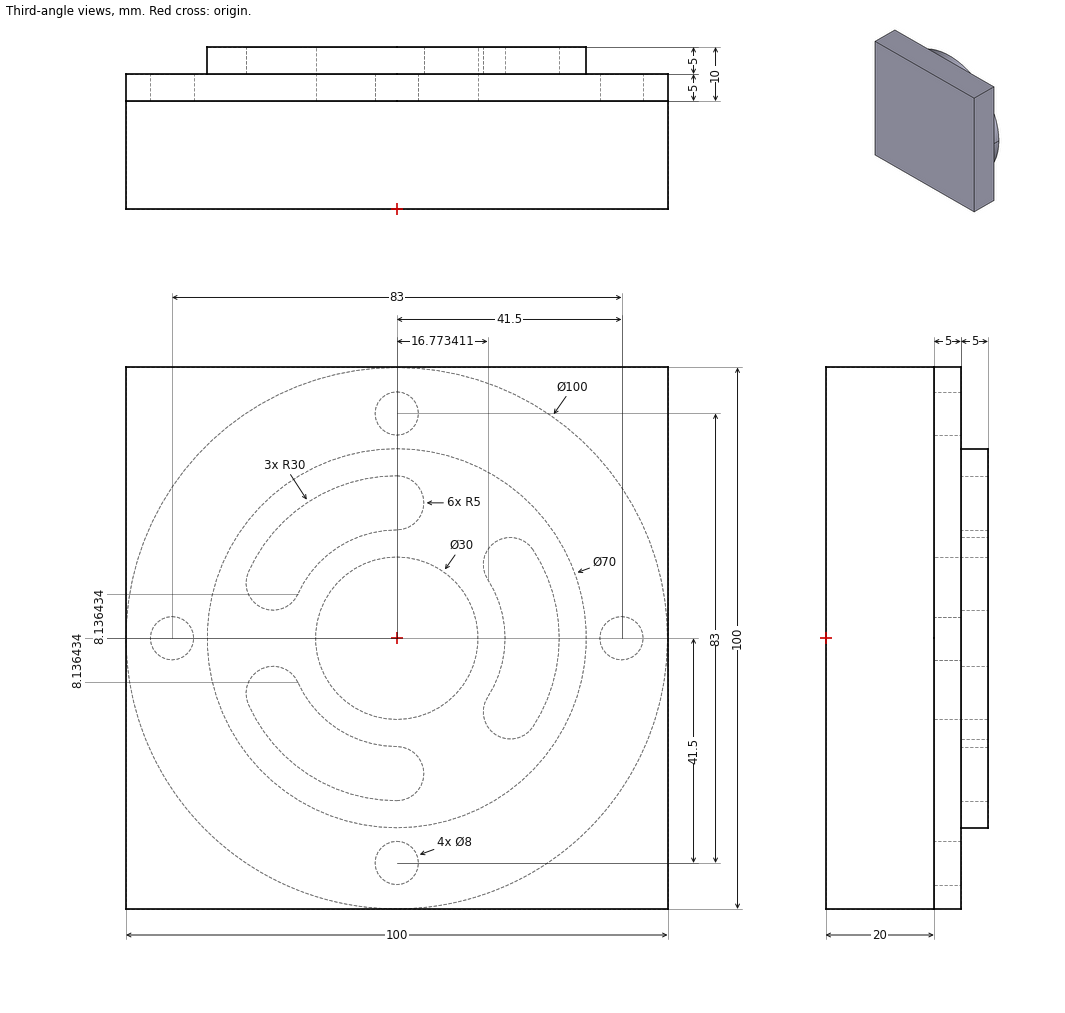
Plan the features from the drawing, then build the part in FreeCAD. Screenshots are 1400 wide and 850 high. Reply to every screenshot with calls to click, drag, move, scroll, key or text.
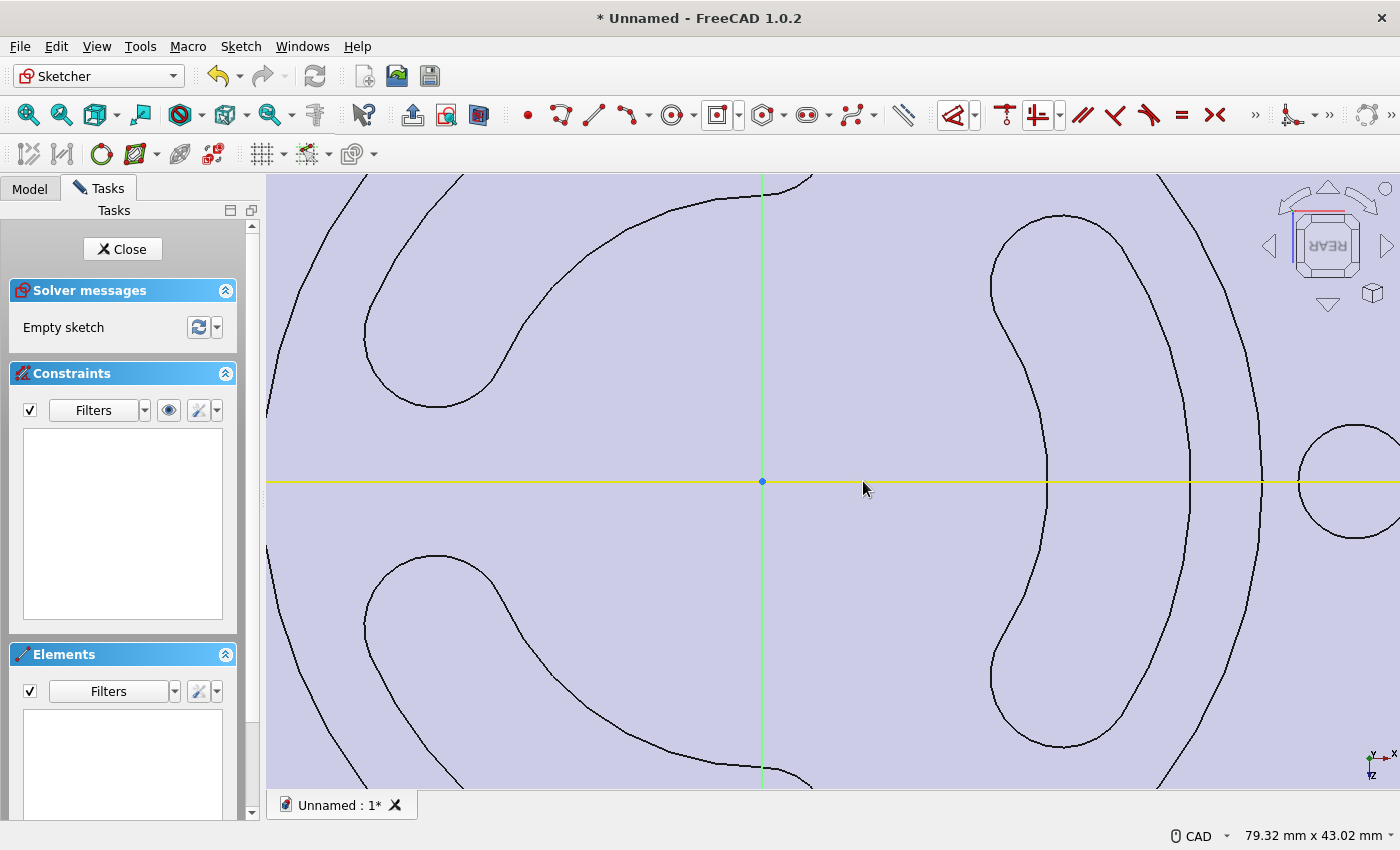
click(672, 116)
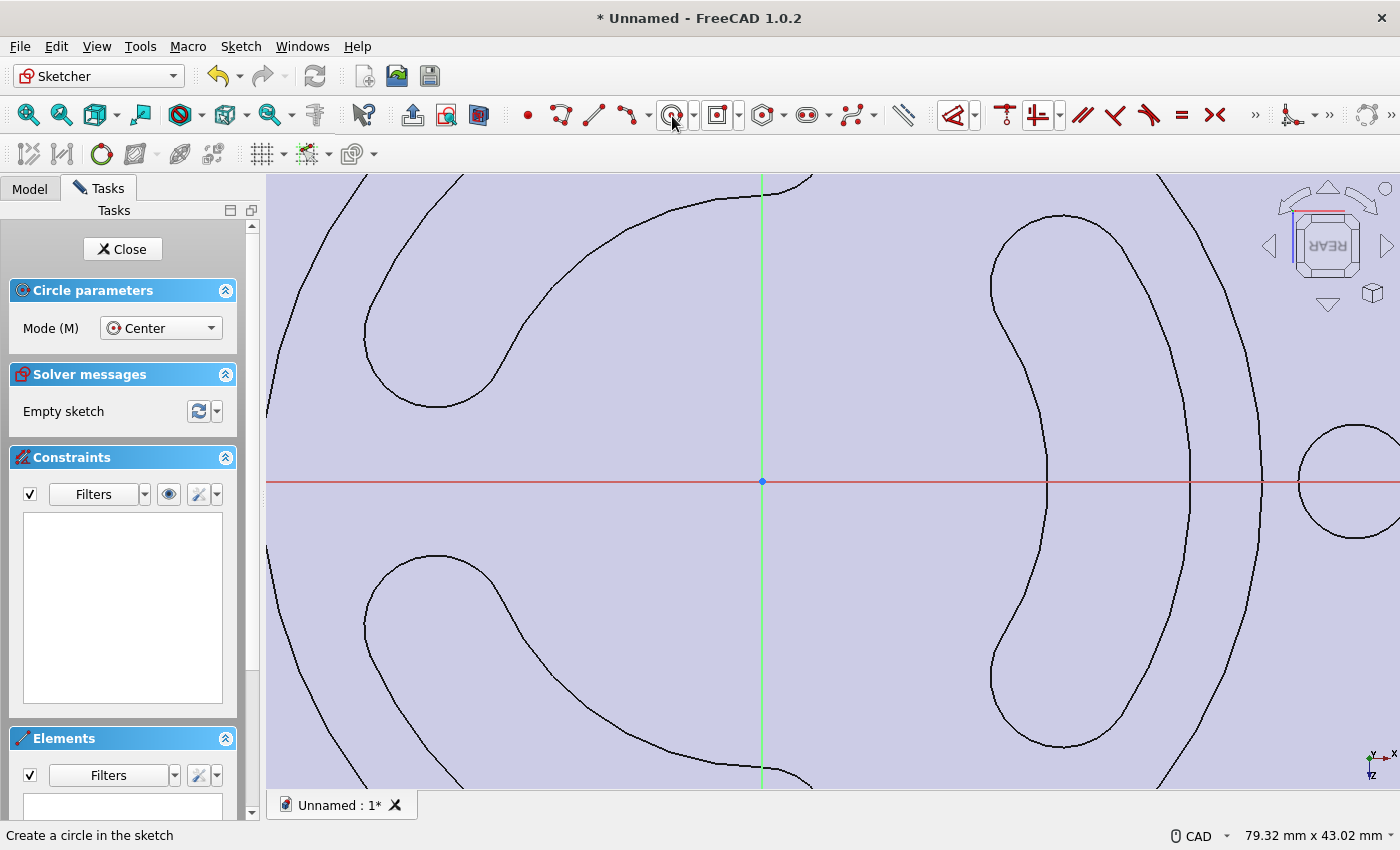
click(762, 481)
move(914, 330)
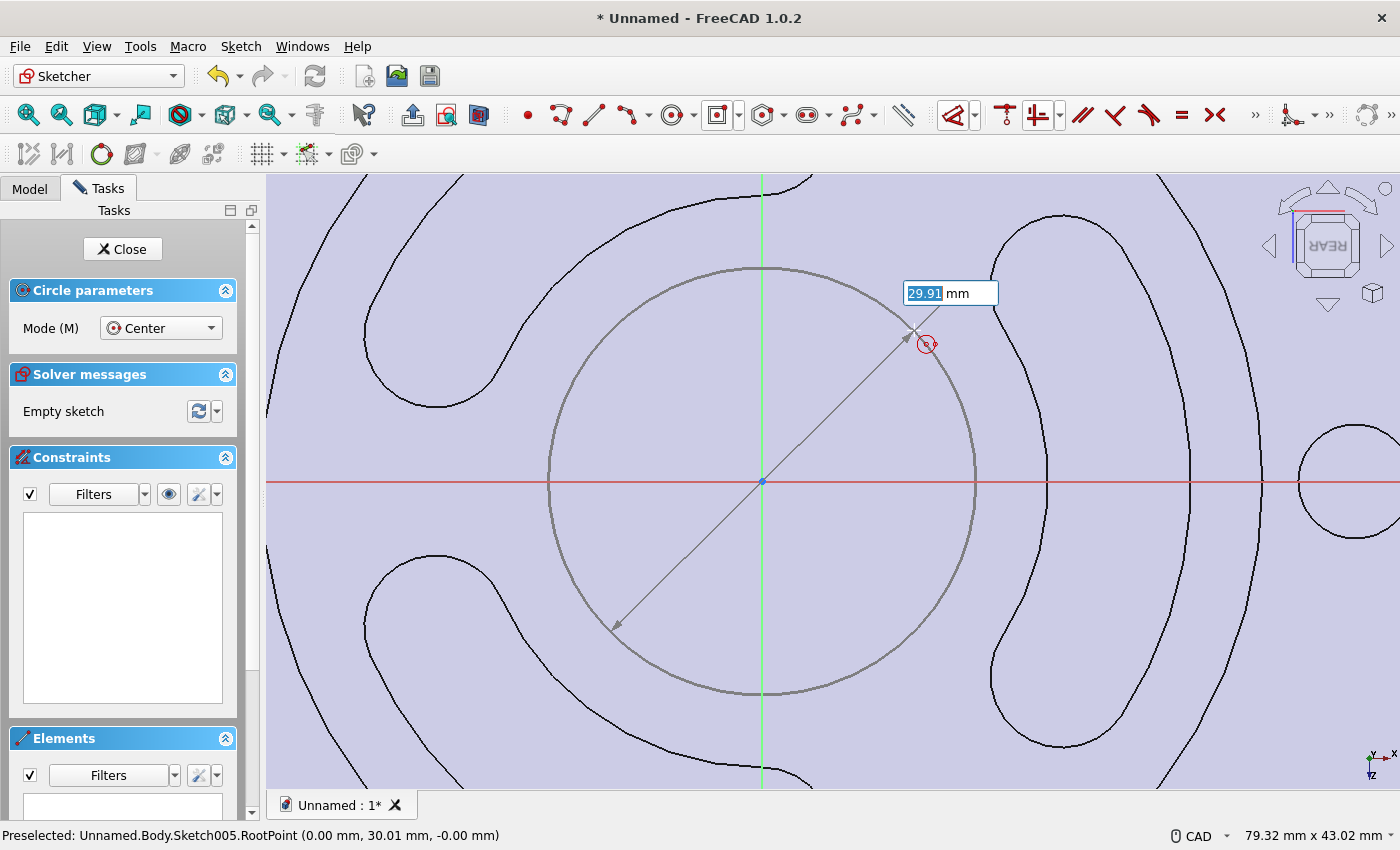
text(30)
key(Return)
key(Escape)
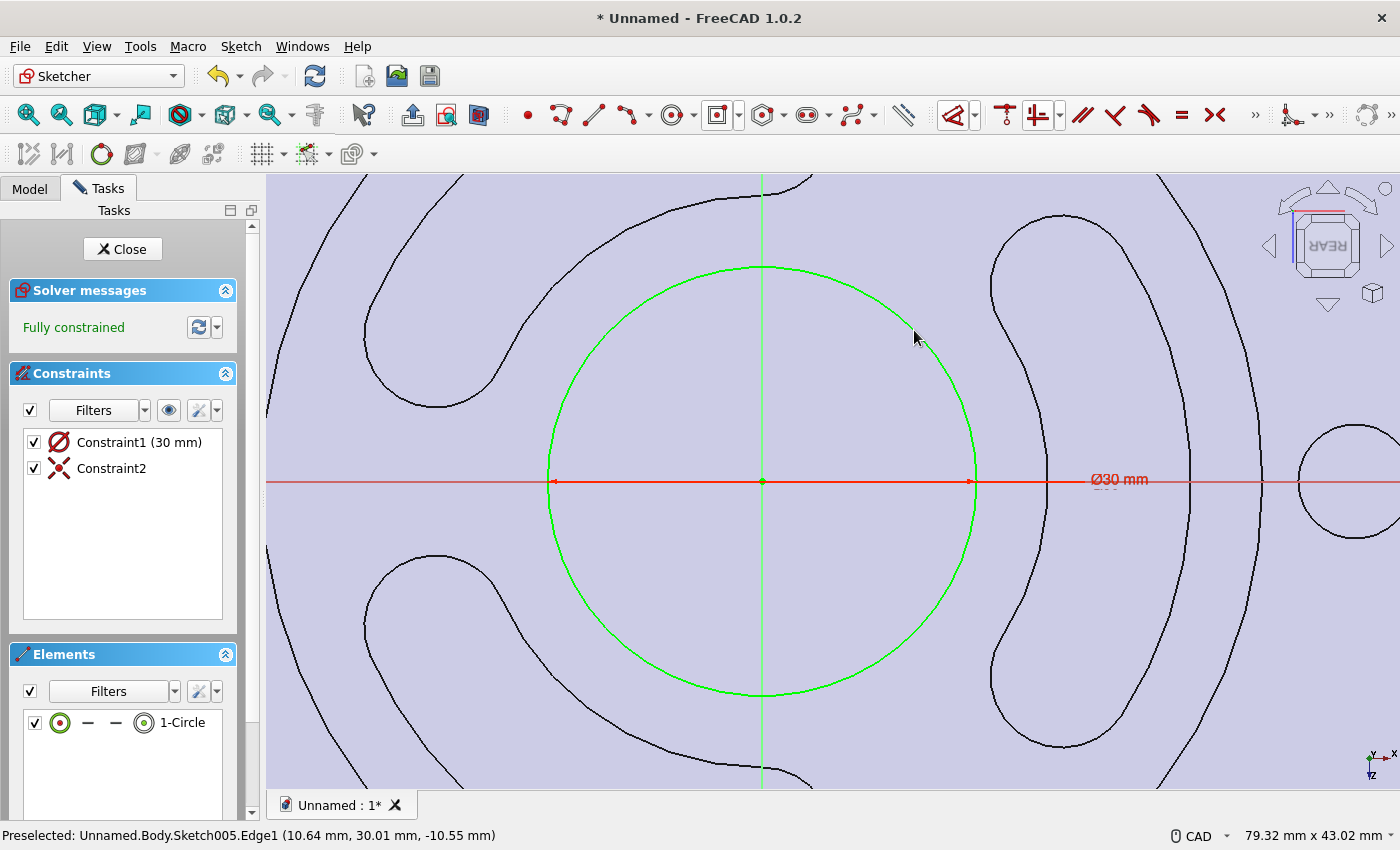
click(123, 249)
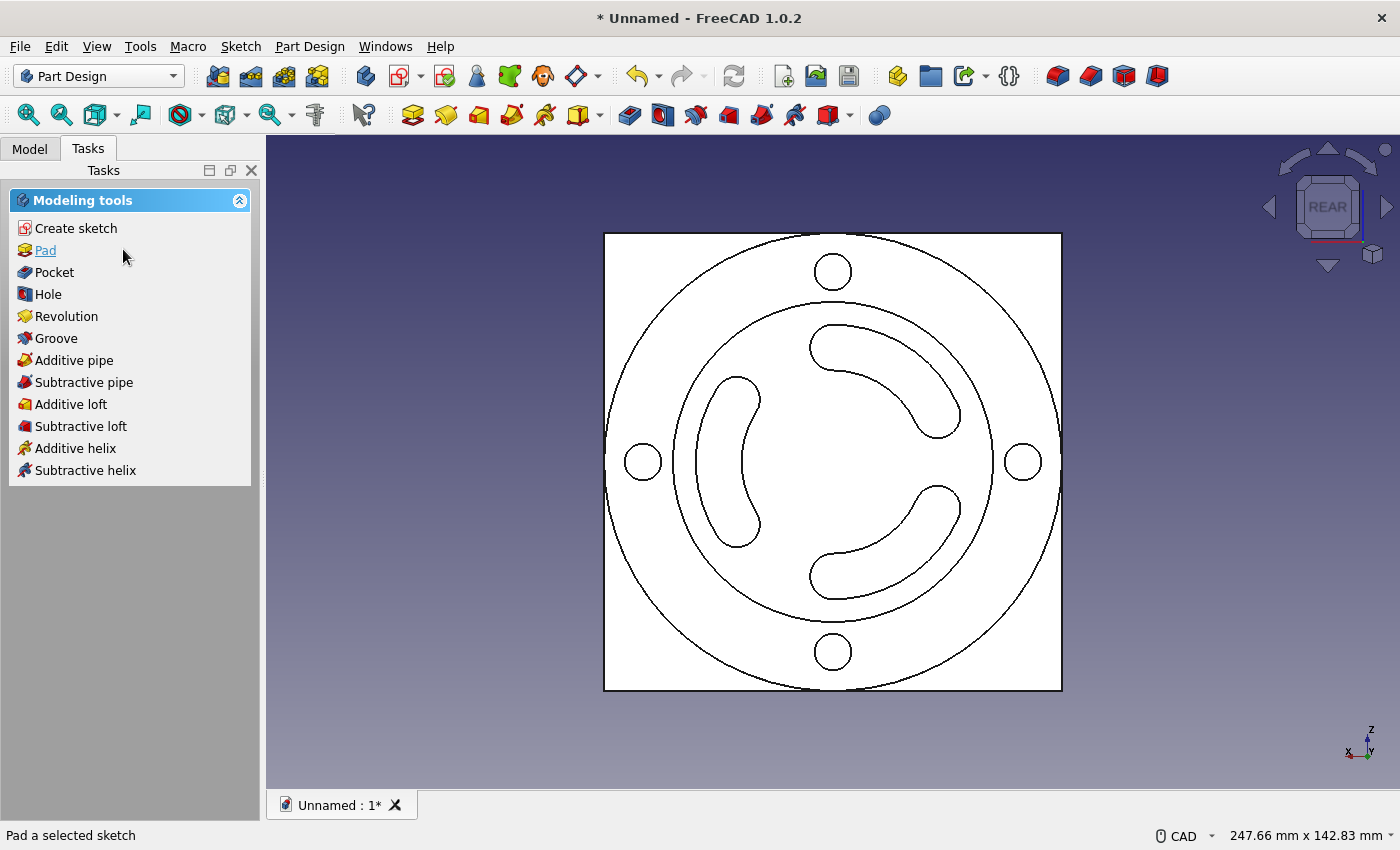
click(630, 116)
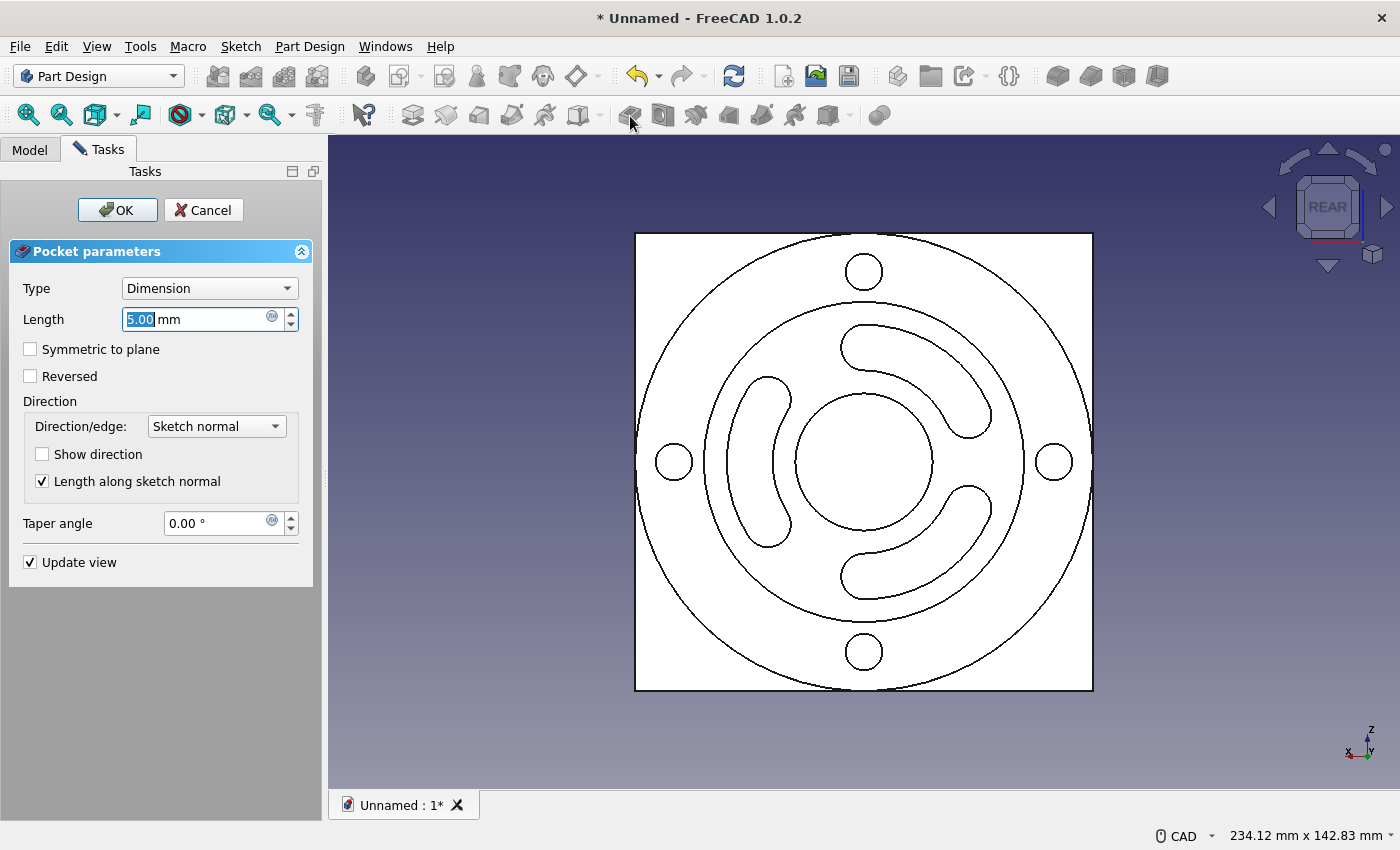
text(10)
key(Tab)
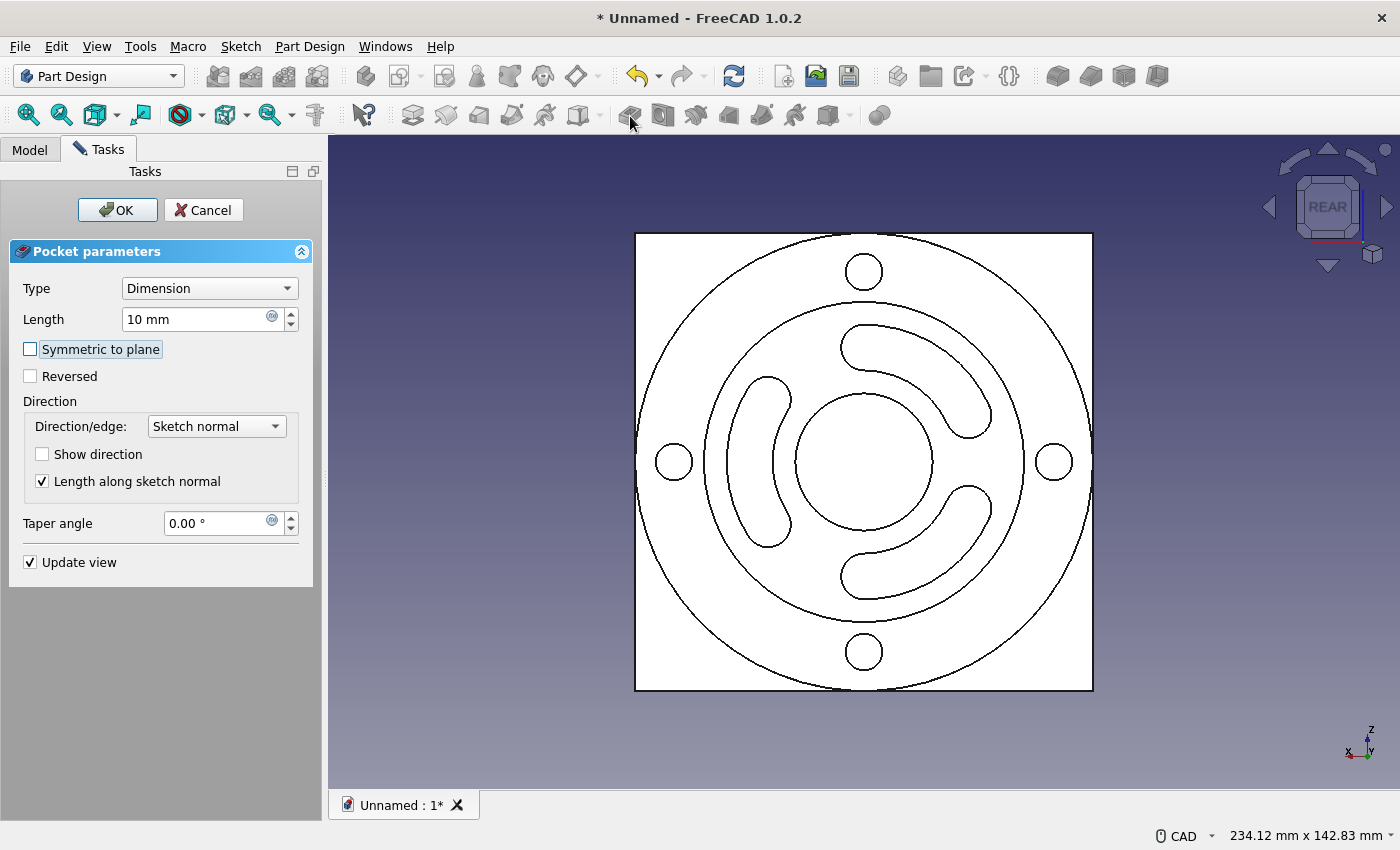
click(118, 210)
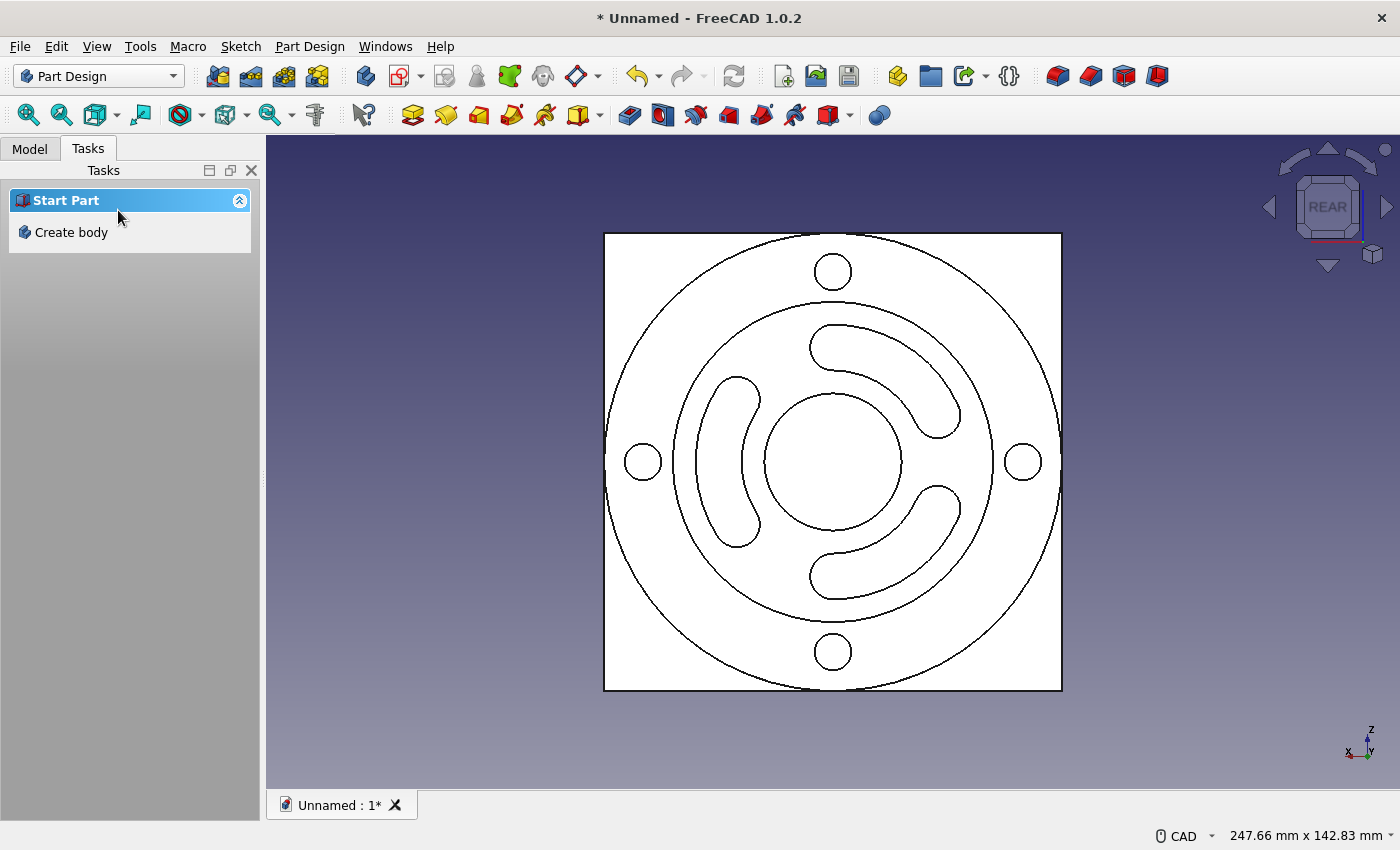
key(0)